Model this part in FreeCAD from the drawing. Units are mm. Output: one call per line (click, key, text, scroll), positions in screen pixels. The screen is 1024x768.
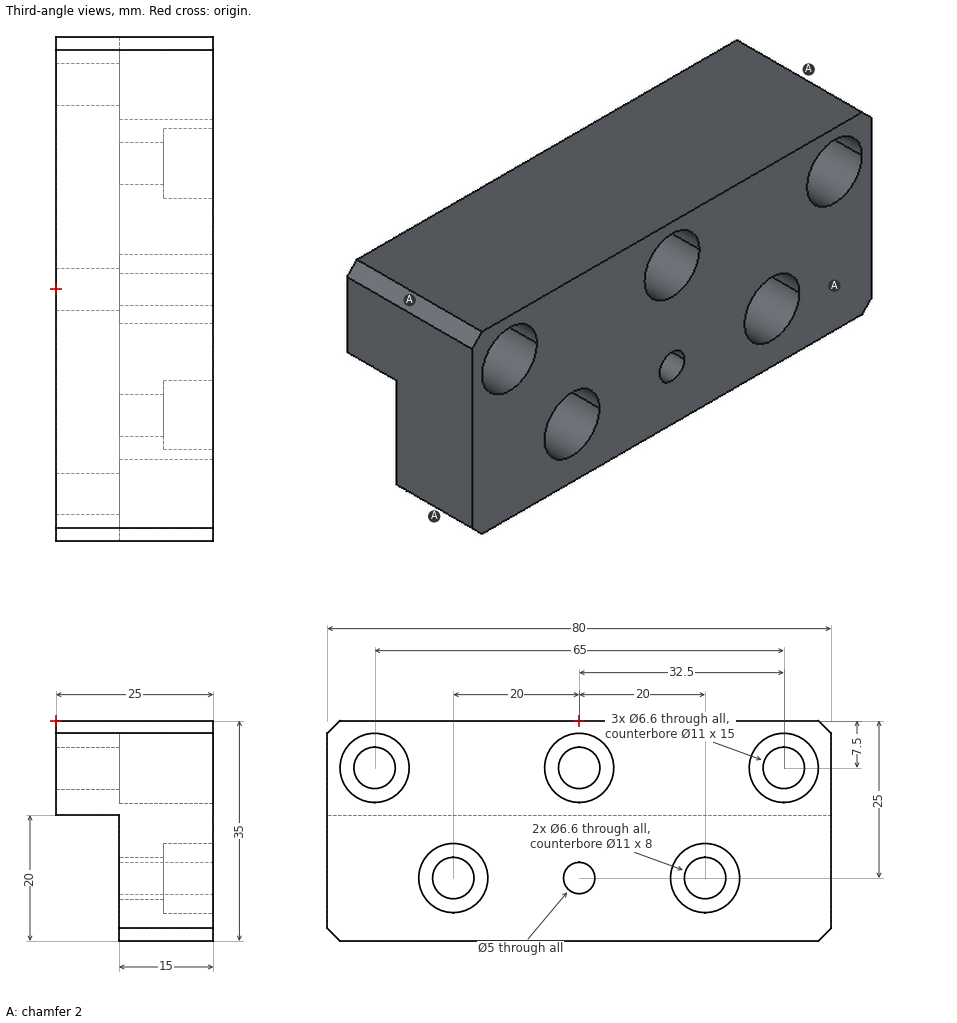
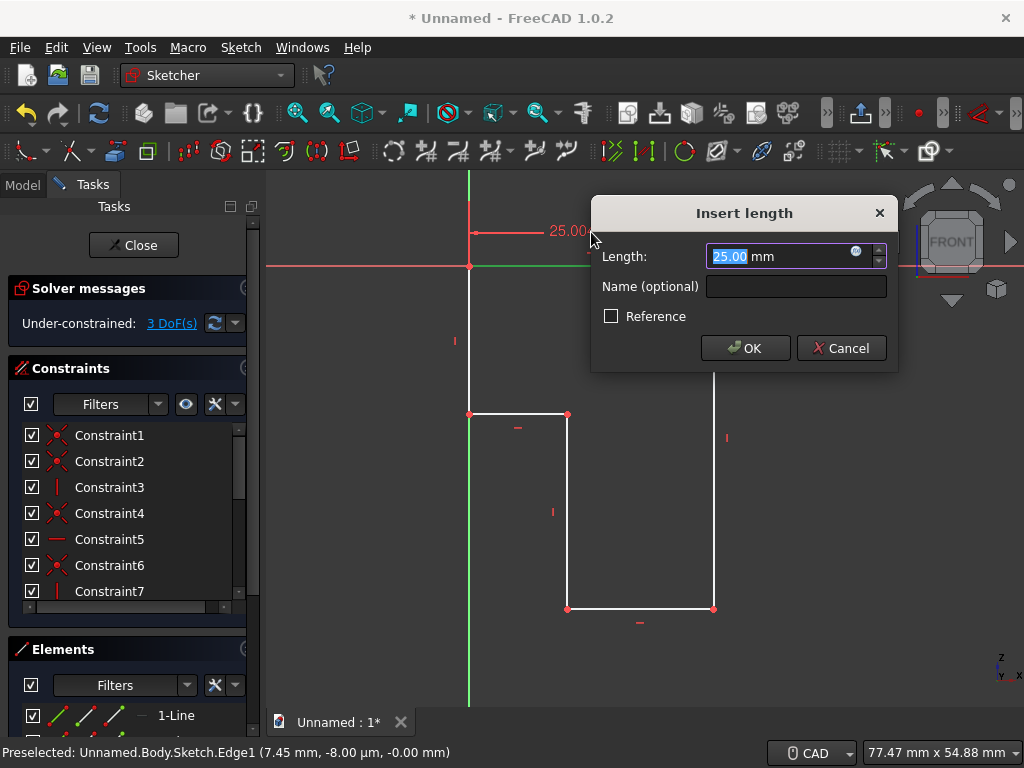
text(25)
key(Return)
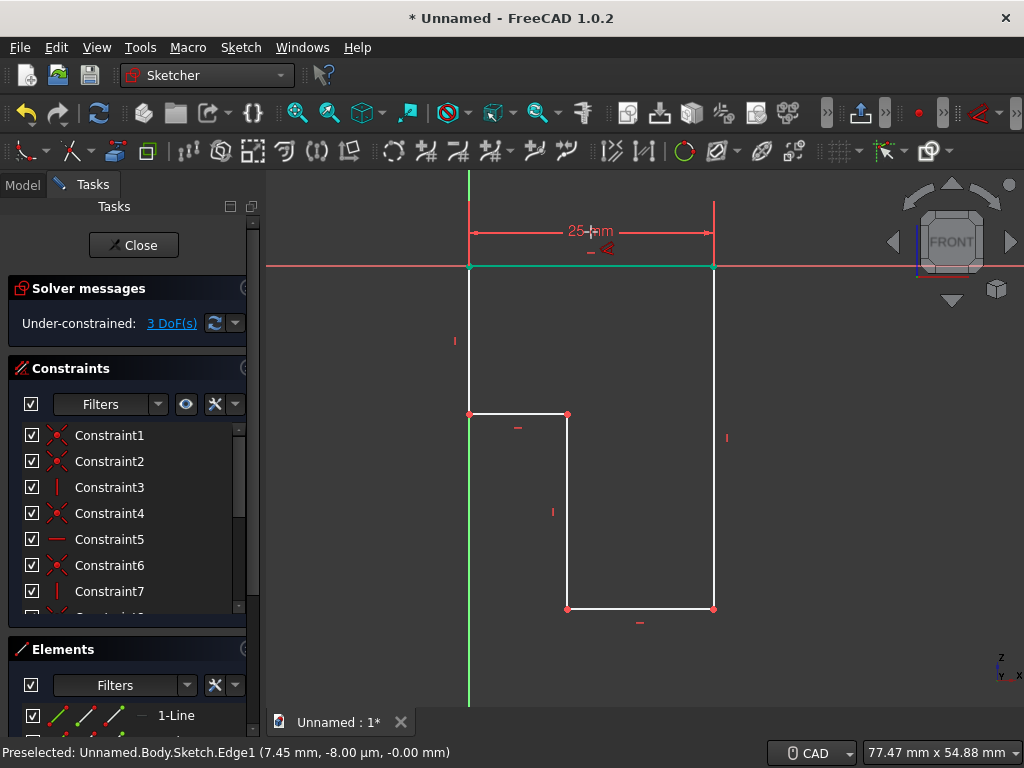
click(714, 369)
click(748, 438)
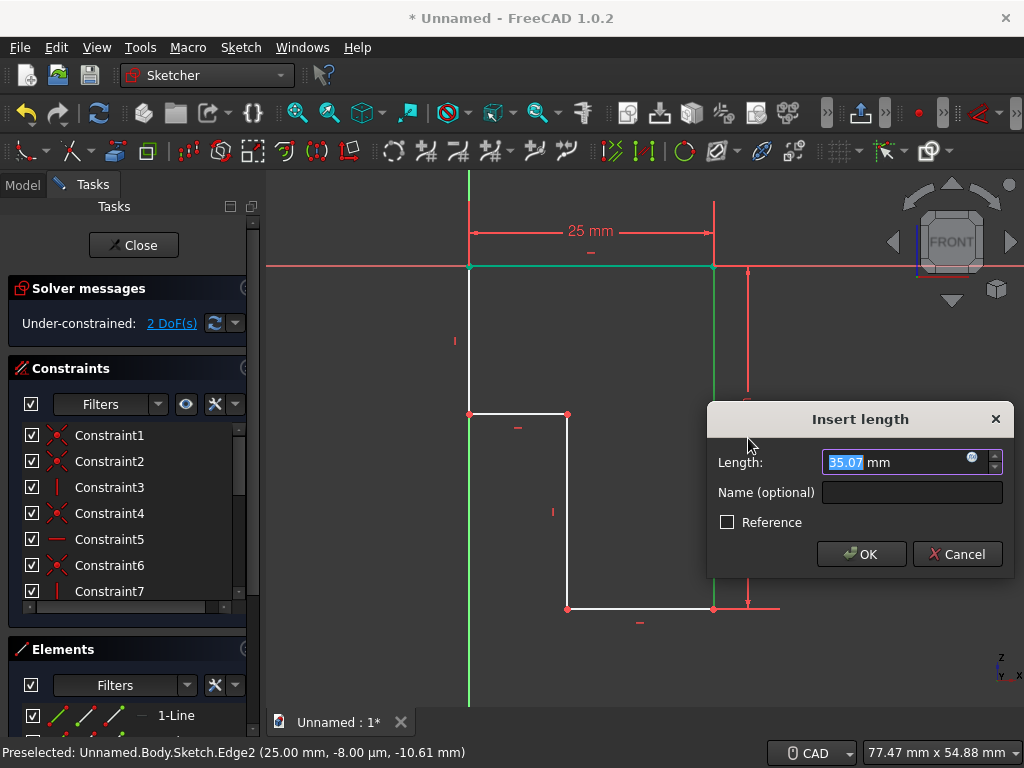
text(35)
key(Return)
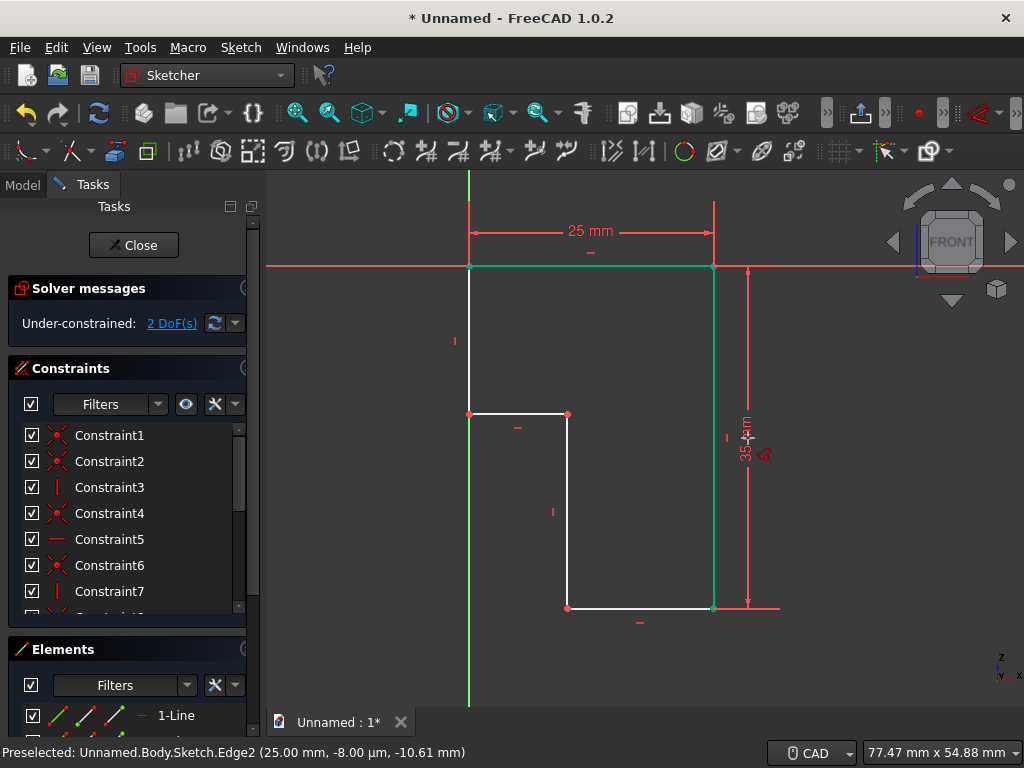
click(670, 609)
click(640, 643)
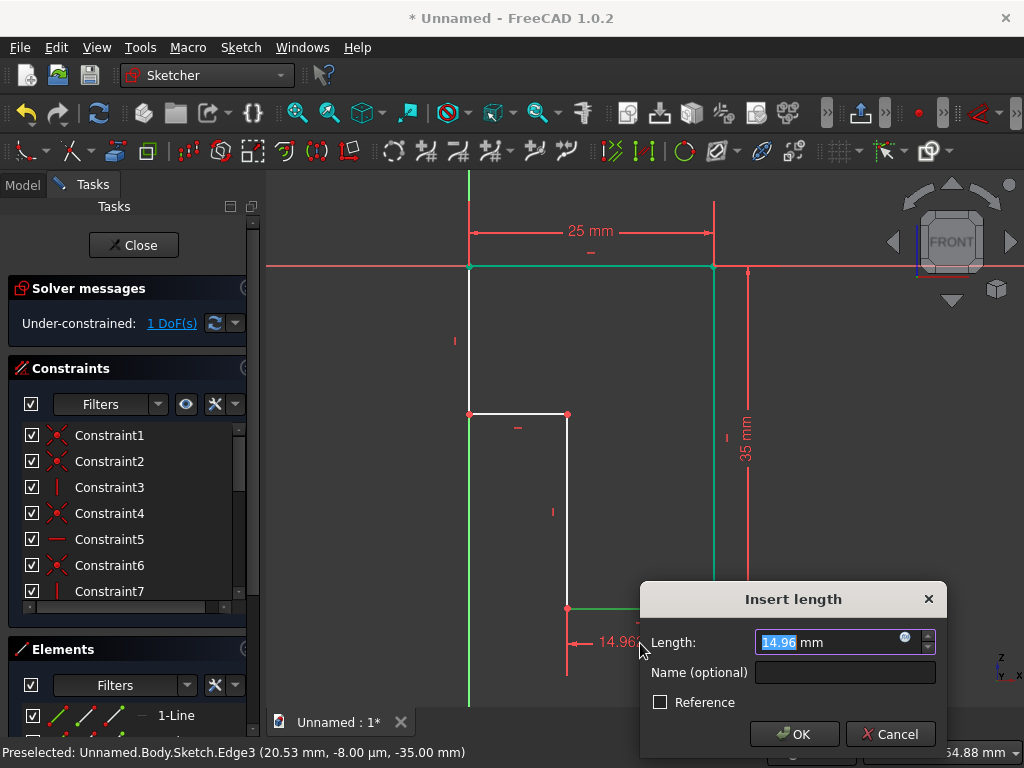
text(15)
key(Return)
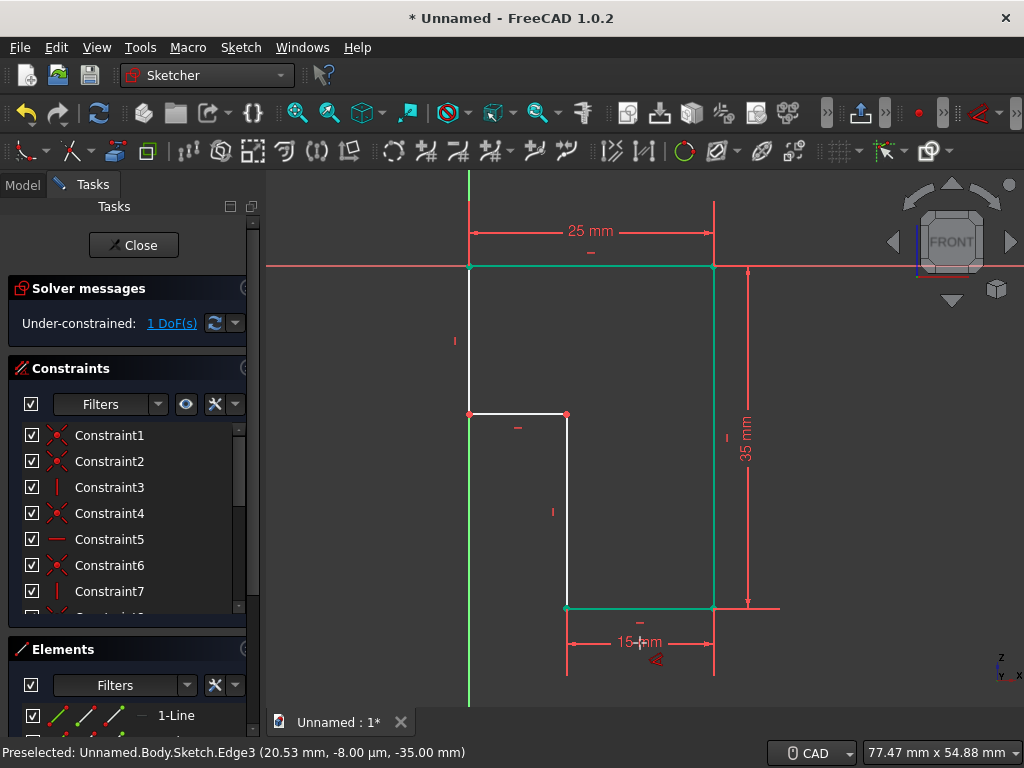
click(567, 550)
click(533, 511)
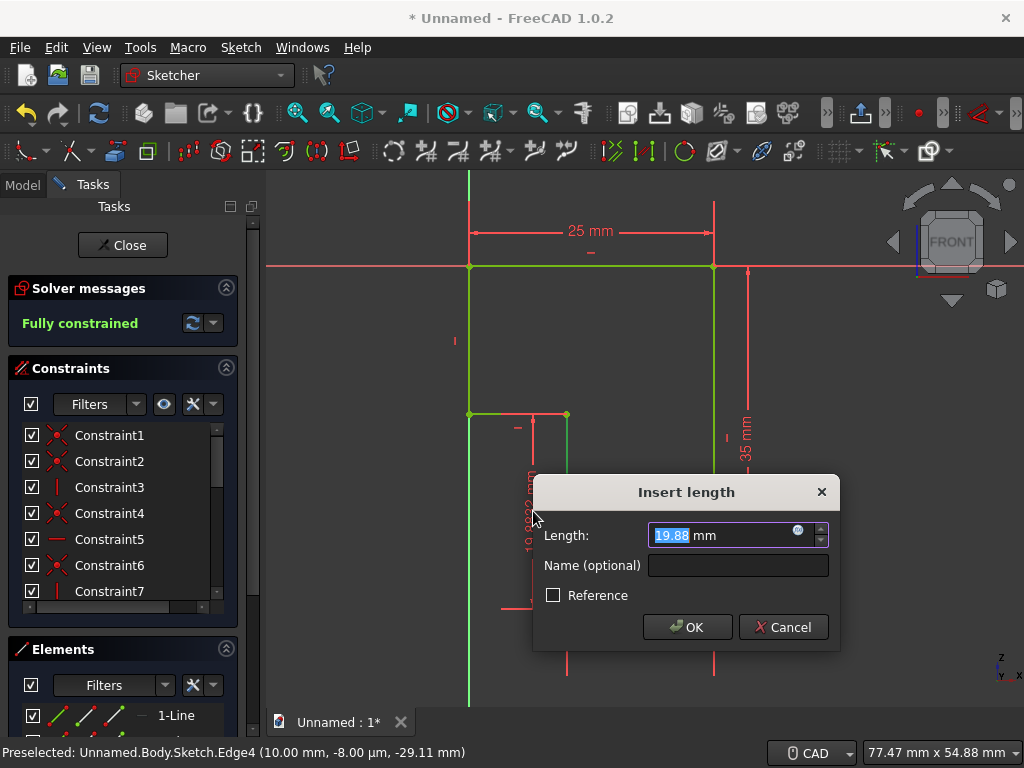
text(20)
key(Return)
key(Escape)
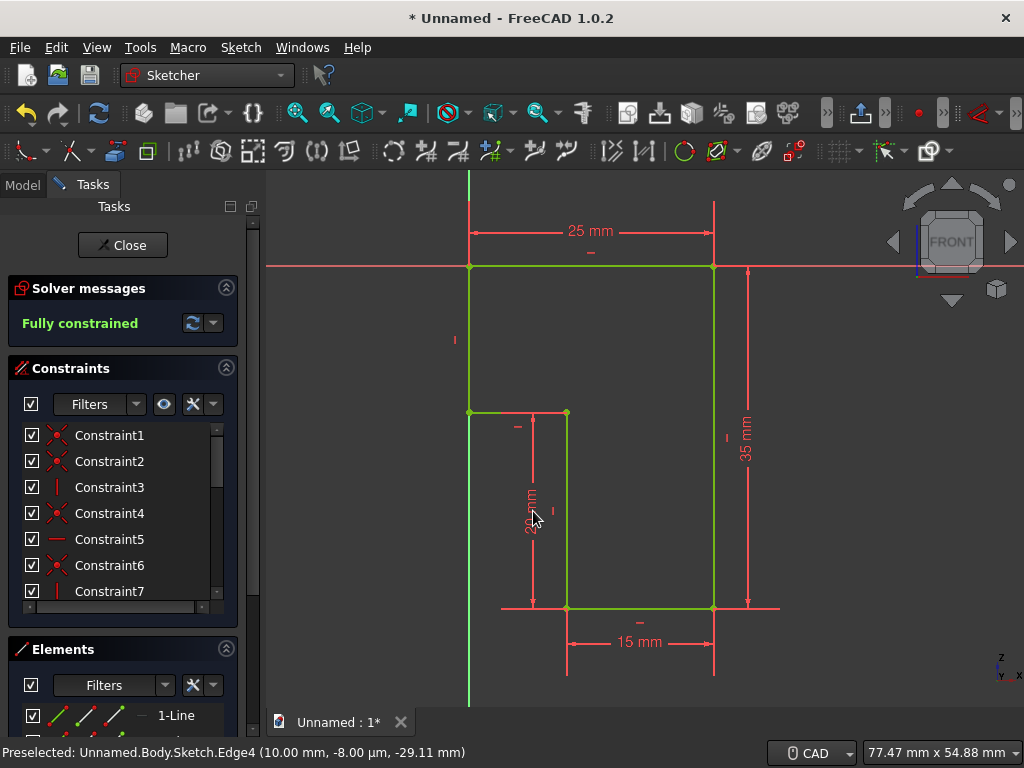
click(123, 245)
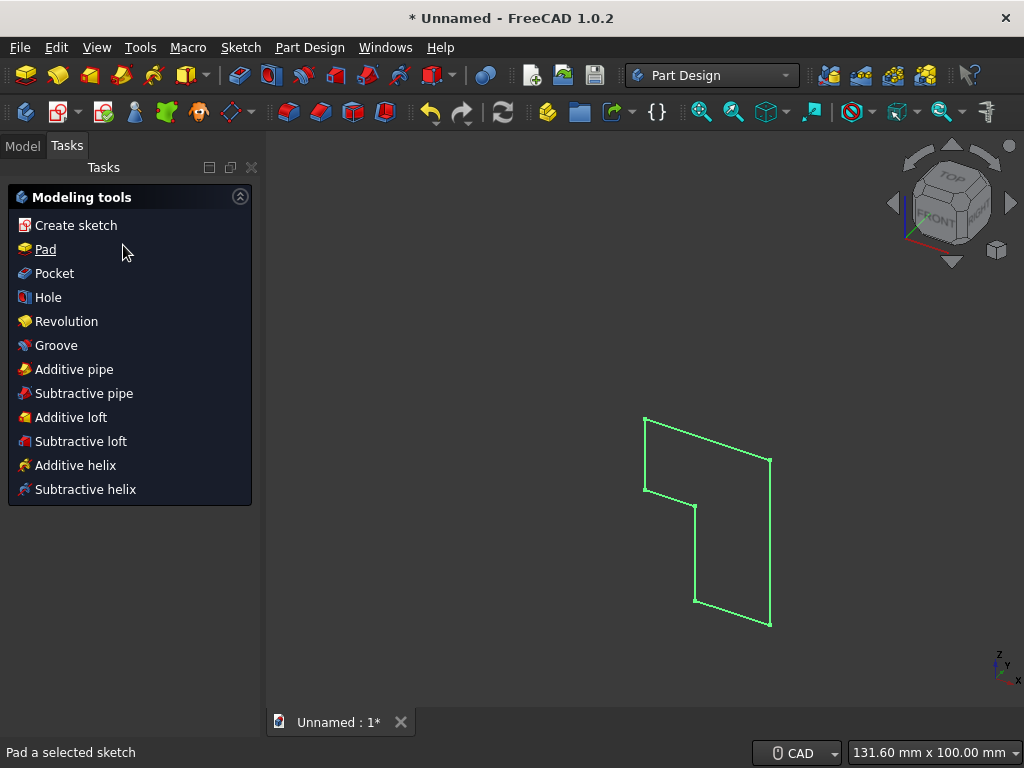
click(26, 76)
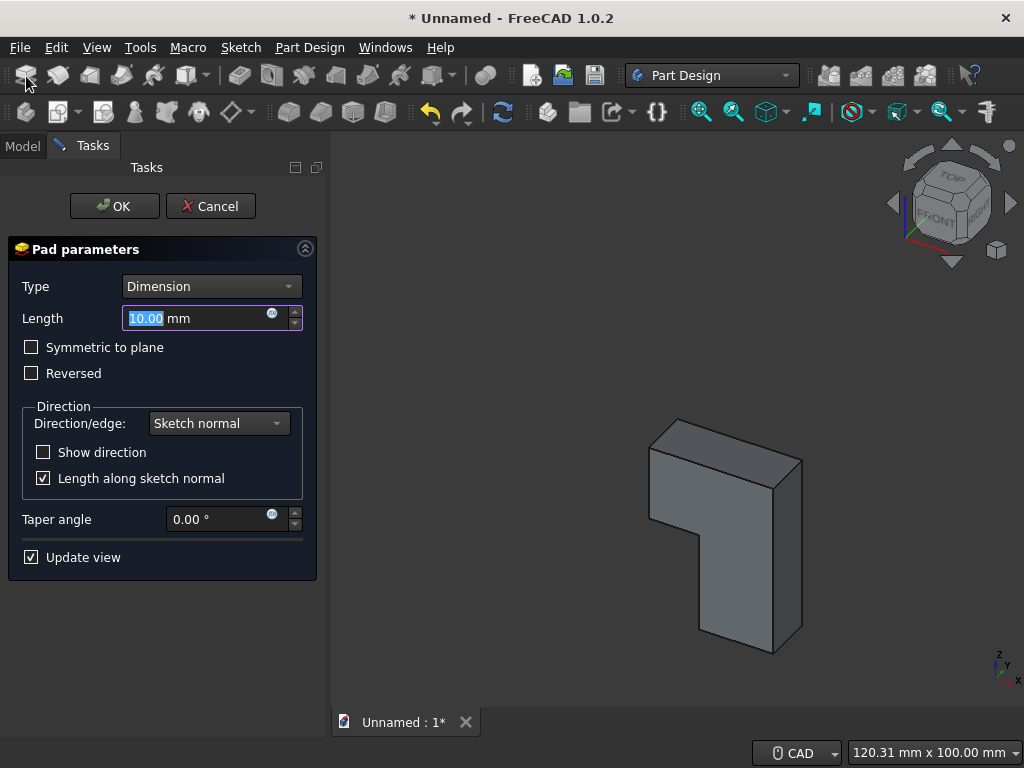
text(80)
key(Tab)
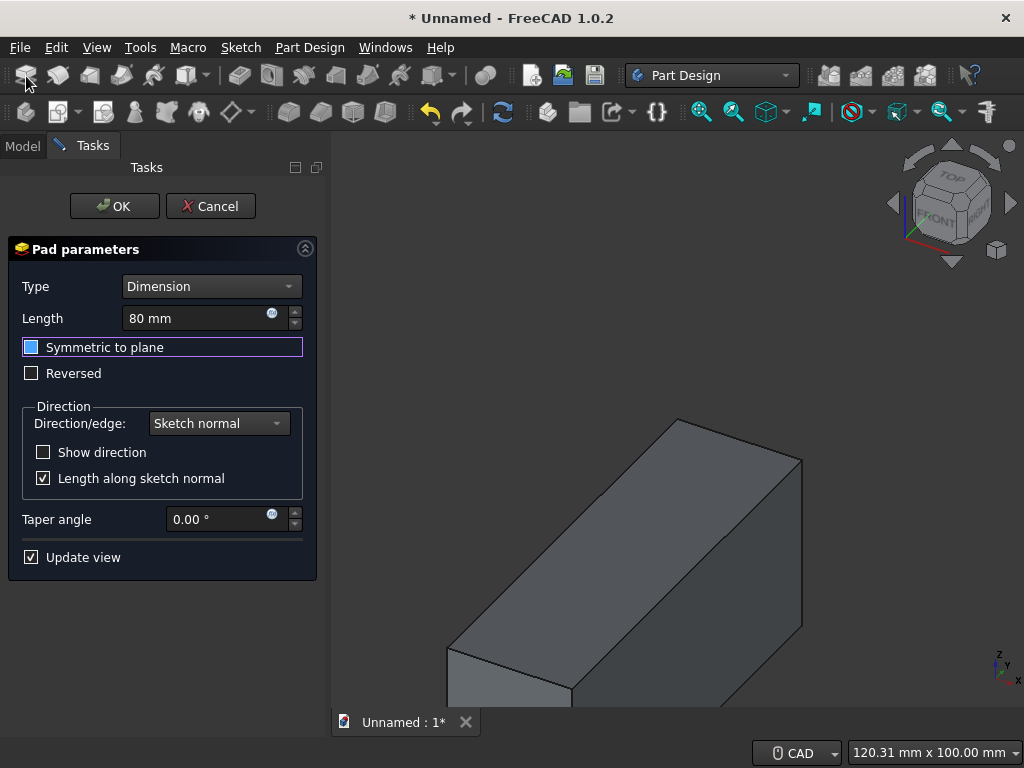
click(30, 347)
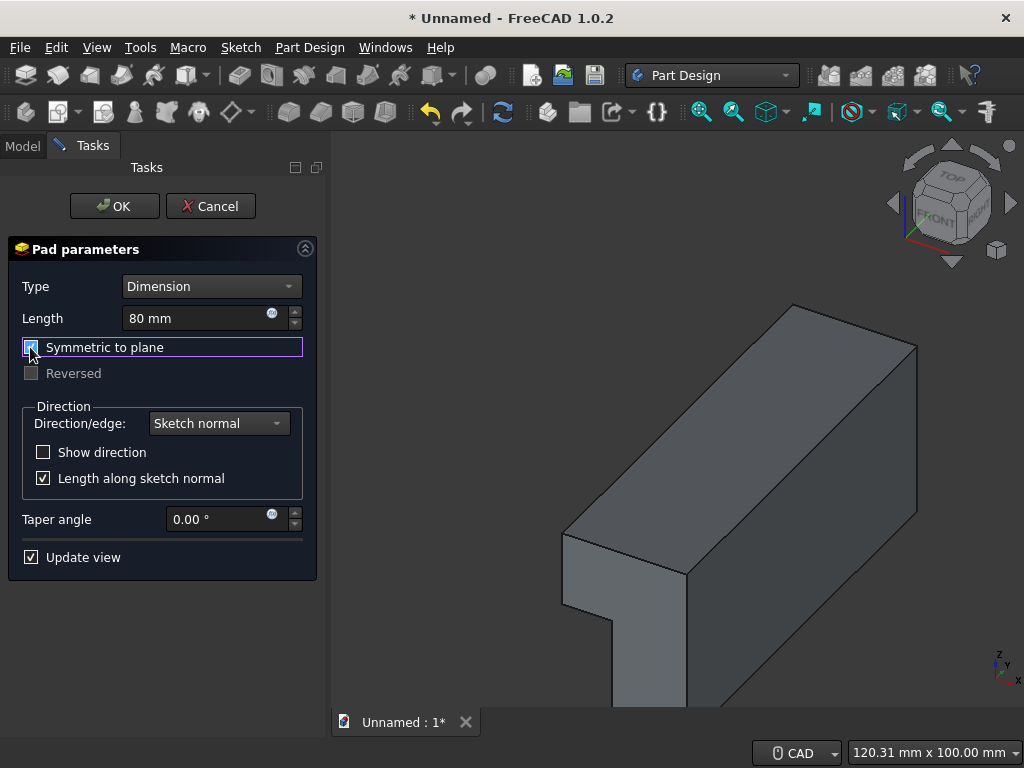
click(115, 206)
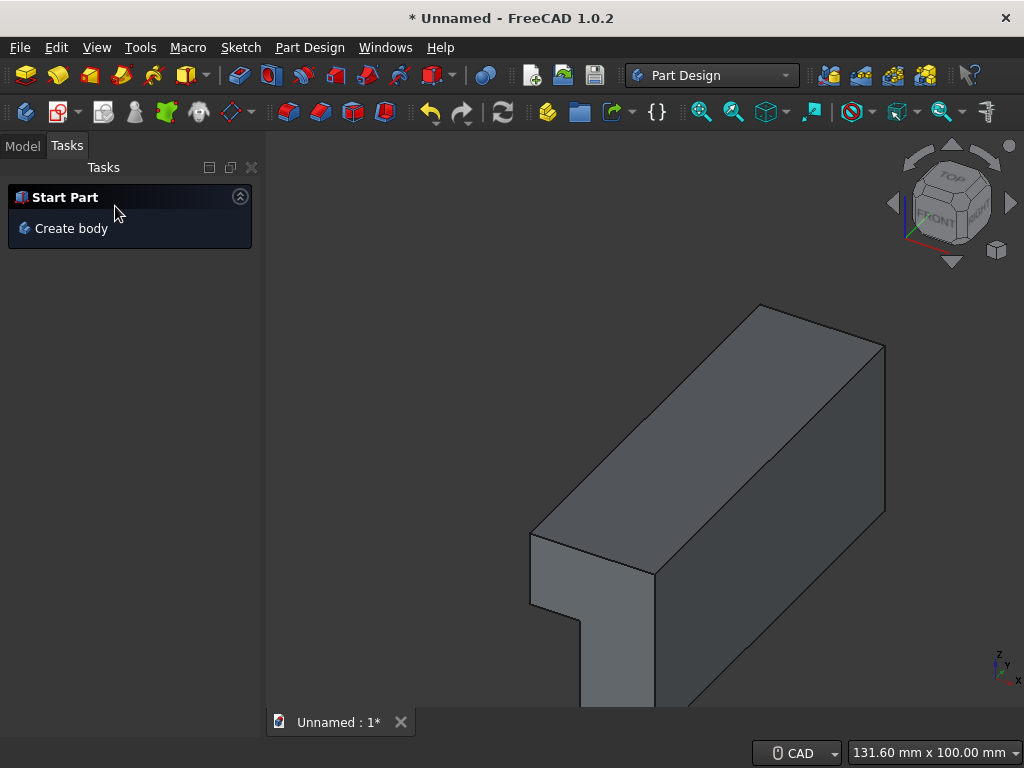
click(702, 112)